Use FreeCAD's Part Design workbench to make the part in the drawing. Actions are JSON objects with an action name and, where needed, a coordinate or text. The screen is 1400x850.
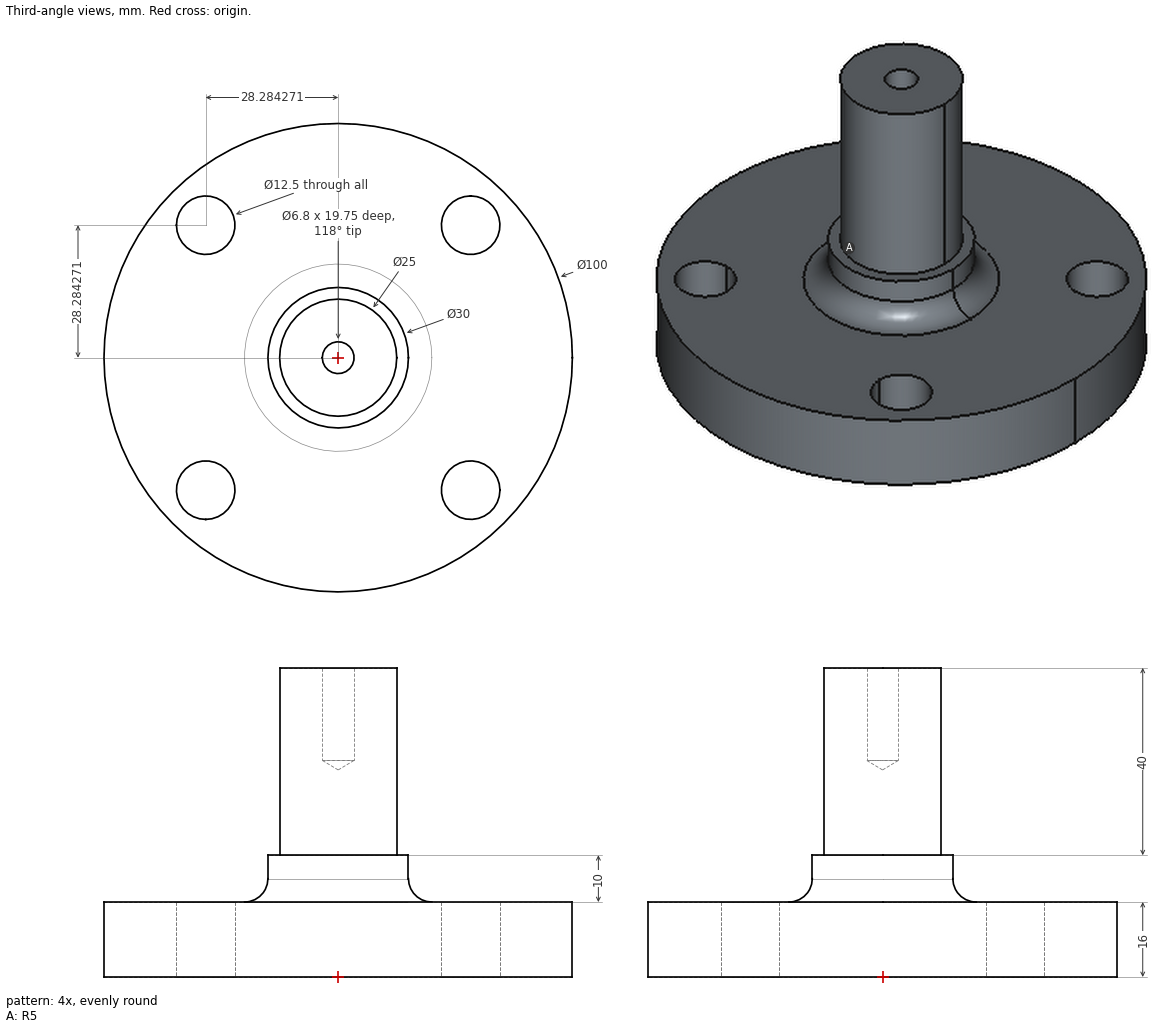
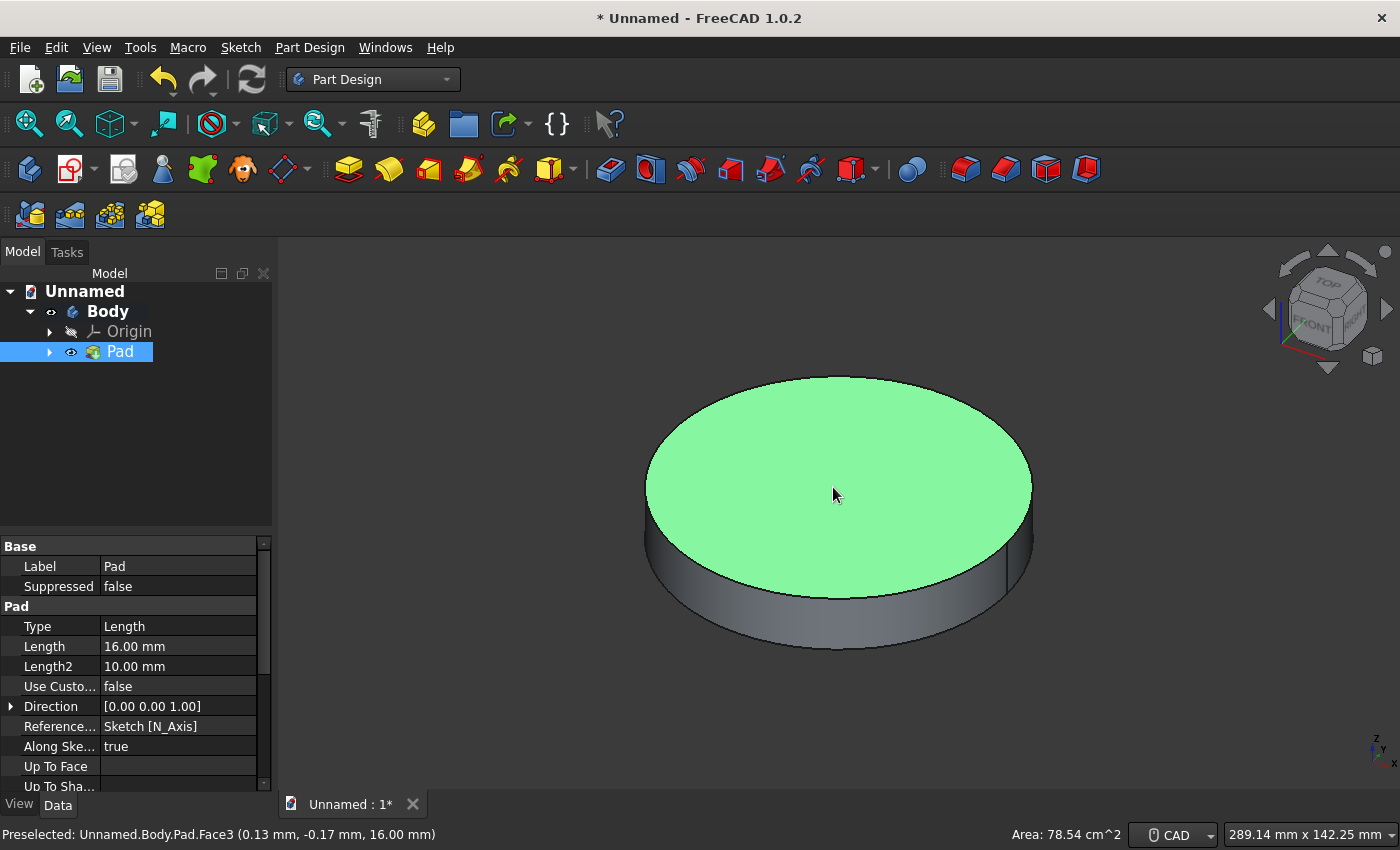
{"action": "left_click", "coordinate": [70, 170]}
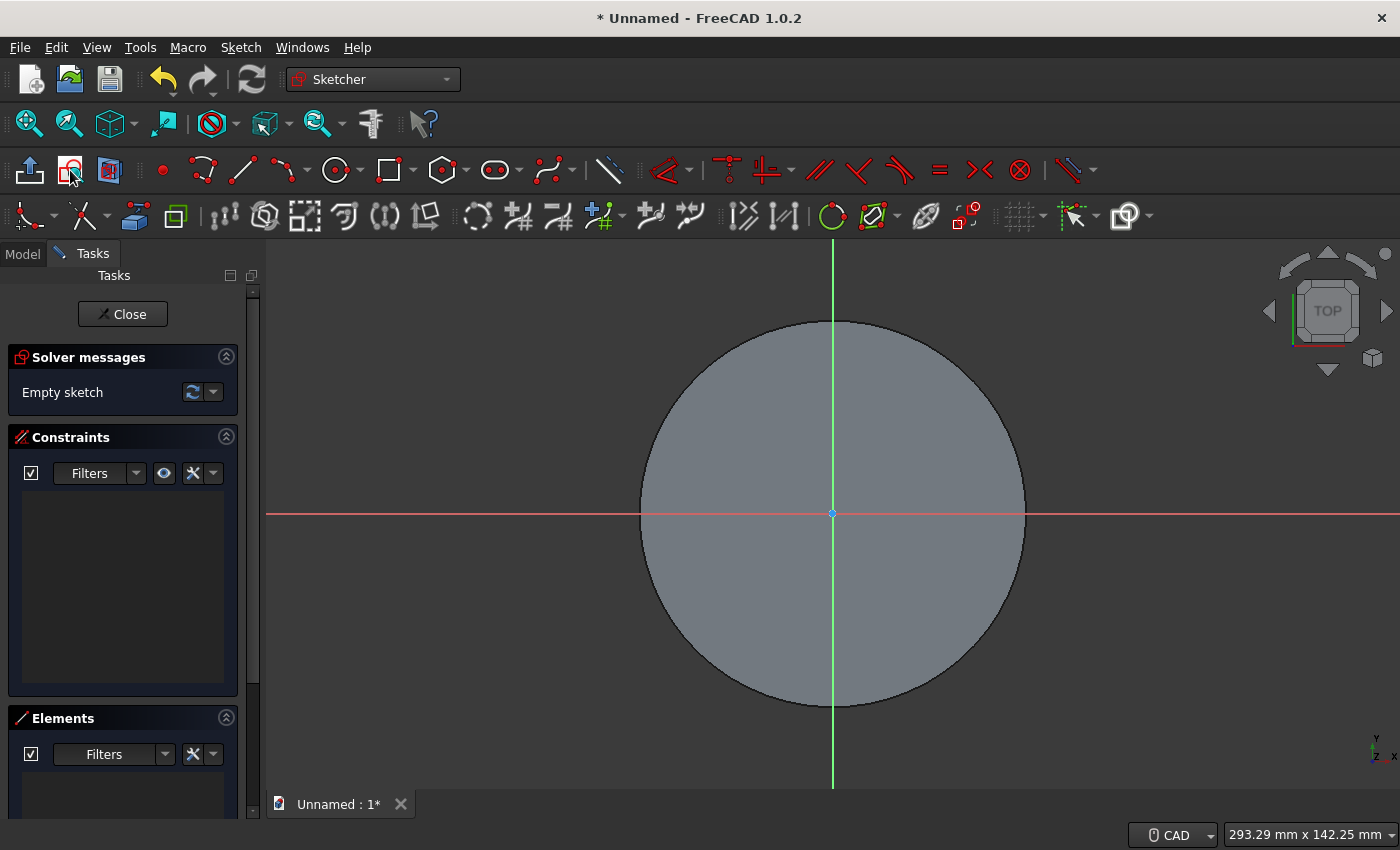
{"action": "scroll", "coordinate": [862, 514], "scroll_direction": "up", "scroll_amount": 6}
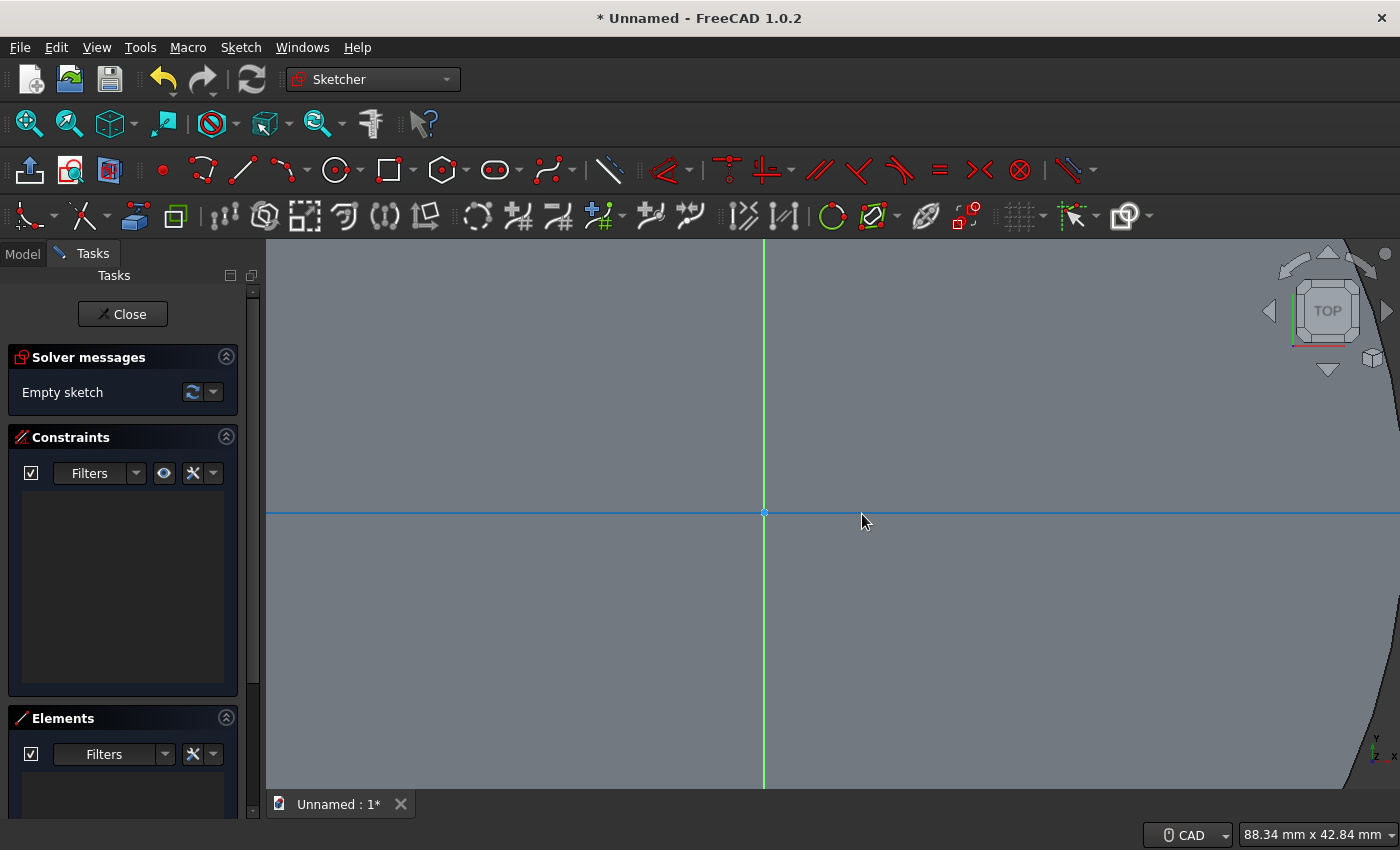
{"action": "key", "text": "g c"}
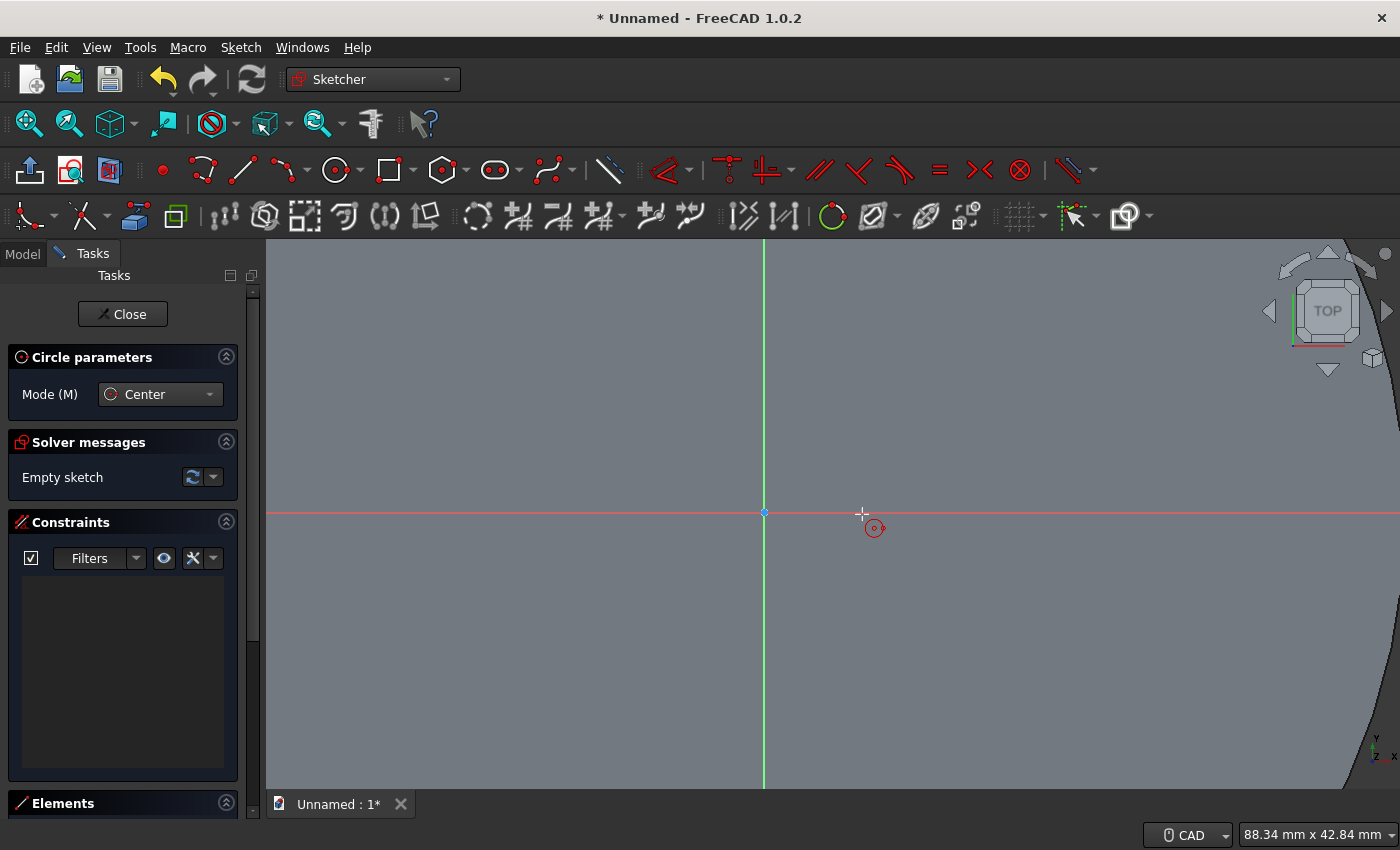
{"action": "left_click", "coordinate": [764, 513]}
{"action": "left_click", "coordinate": [900, 377]}
{"action": "key", "text": "Escape"}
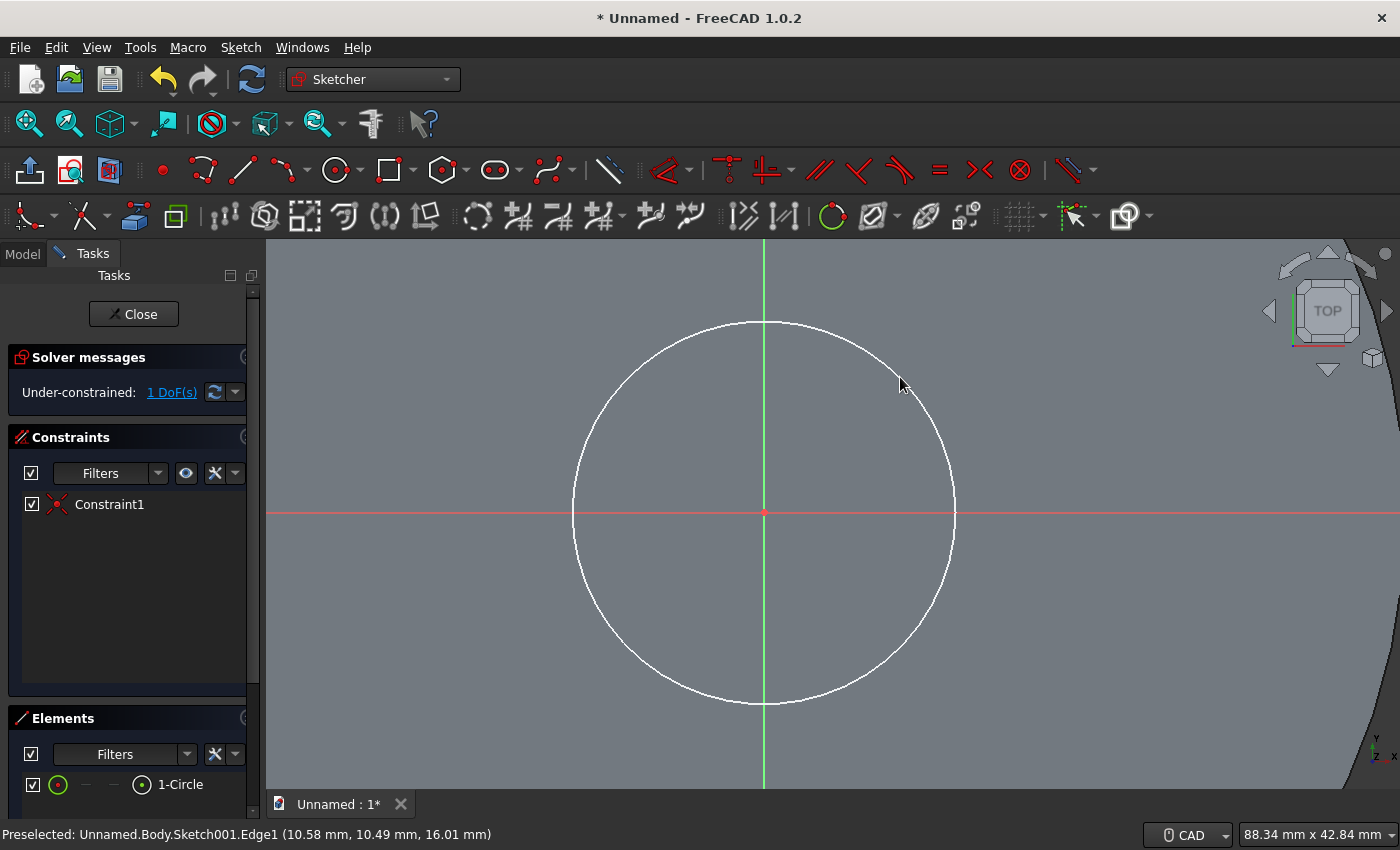
{"action": "left_click", "coordinate": [664, 170]}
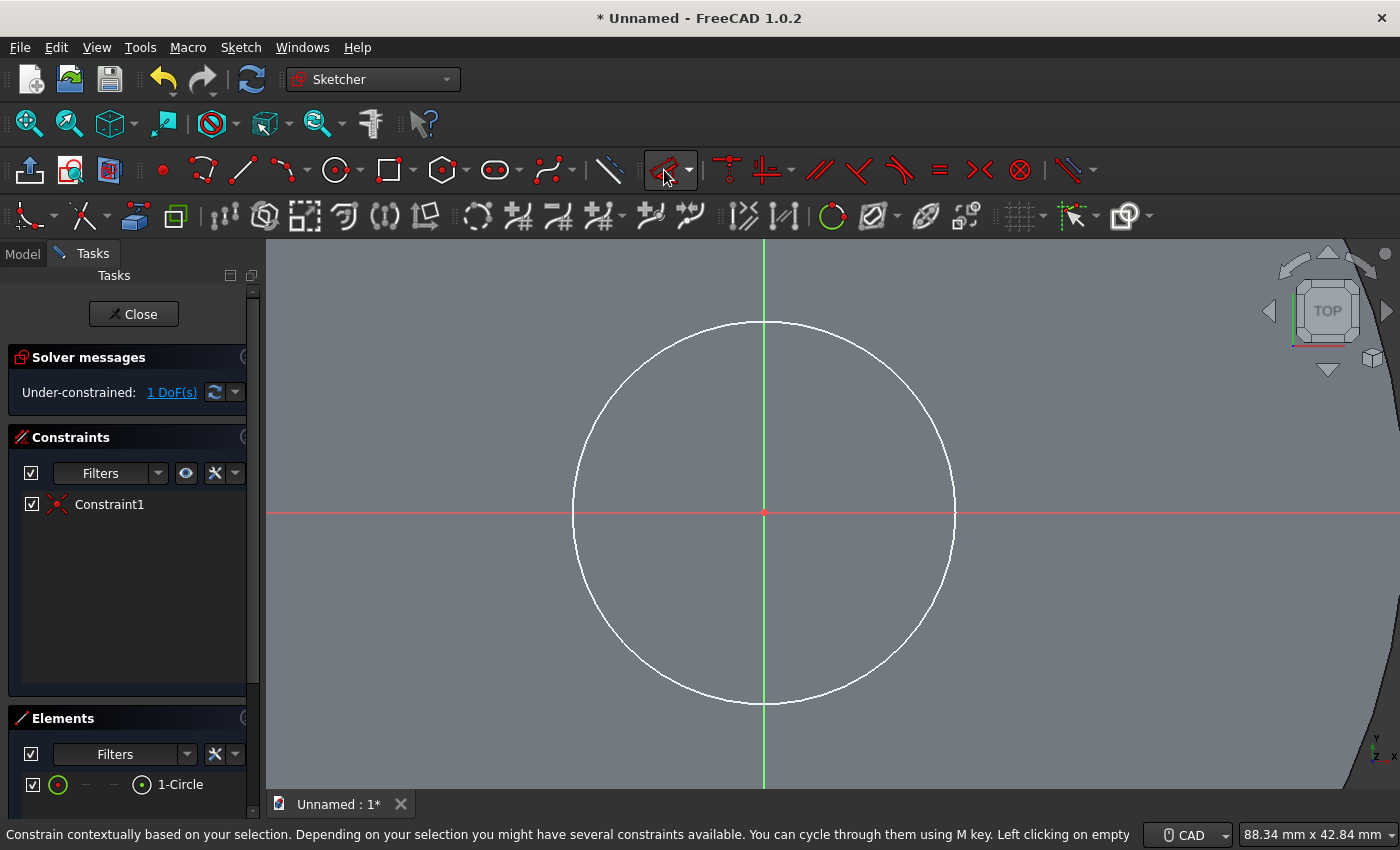
{"action": "left_click", "coordinate": [899, 377]}
{"action": "left_click", "coordinate": [922, 354]}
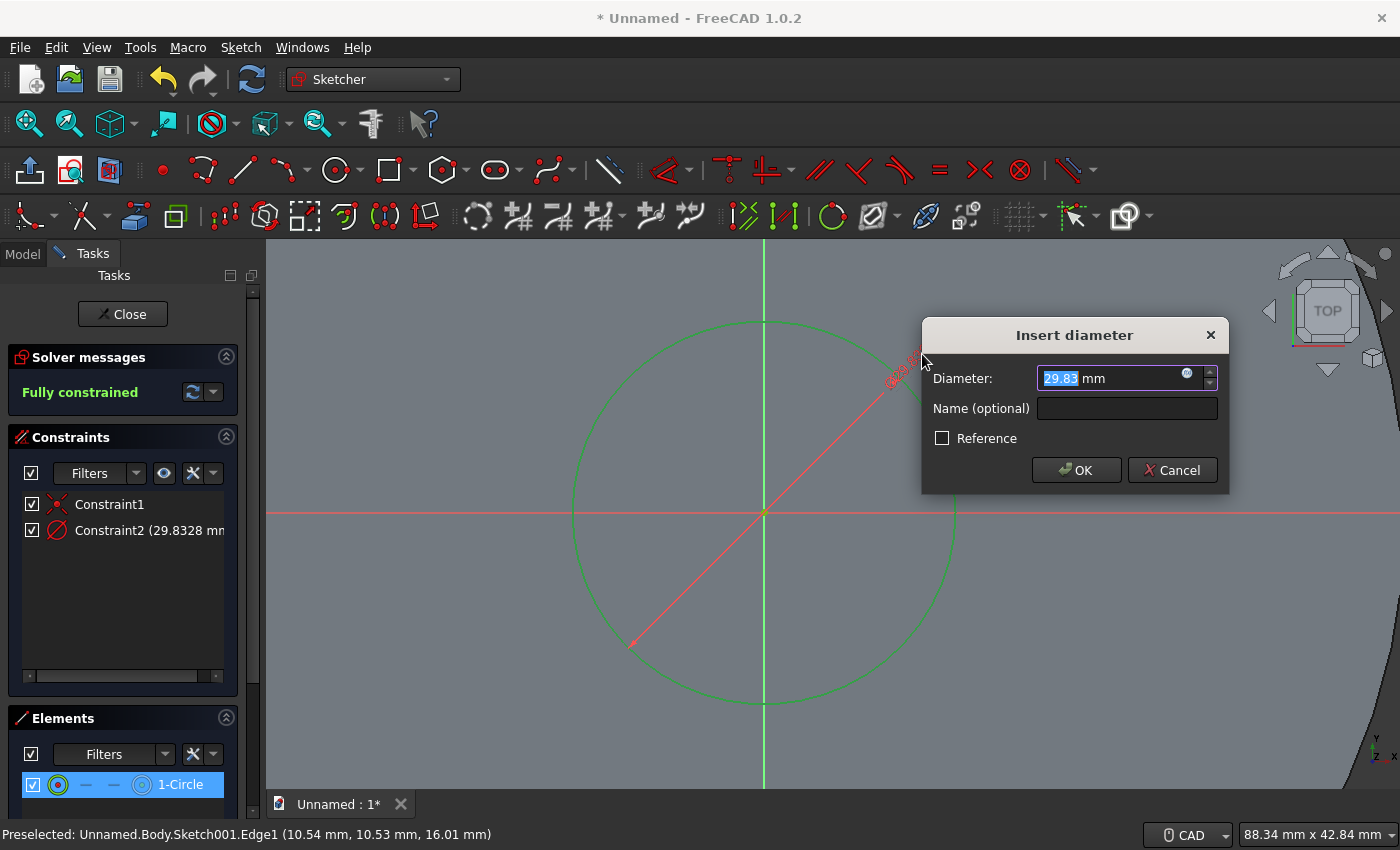
{"action": "type", "text": "30"}
{"action": "key", "text": "Return"}
{"action": "key", "text": "Escape"}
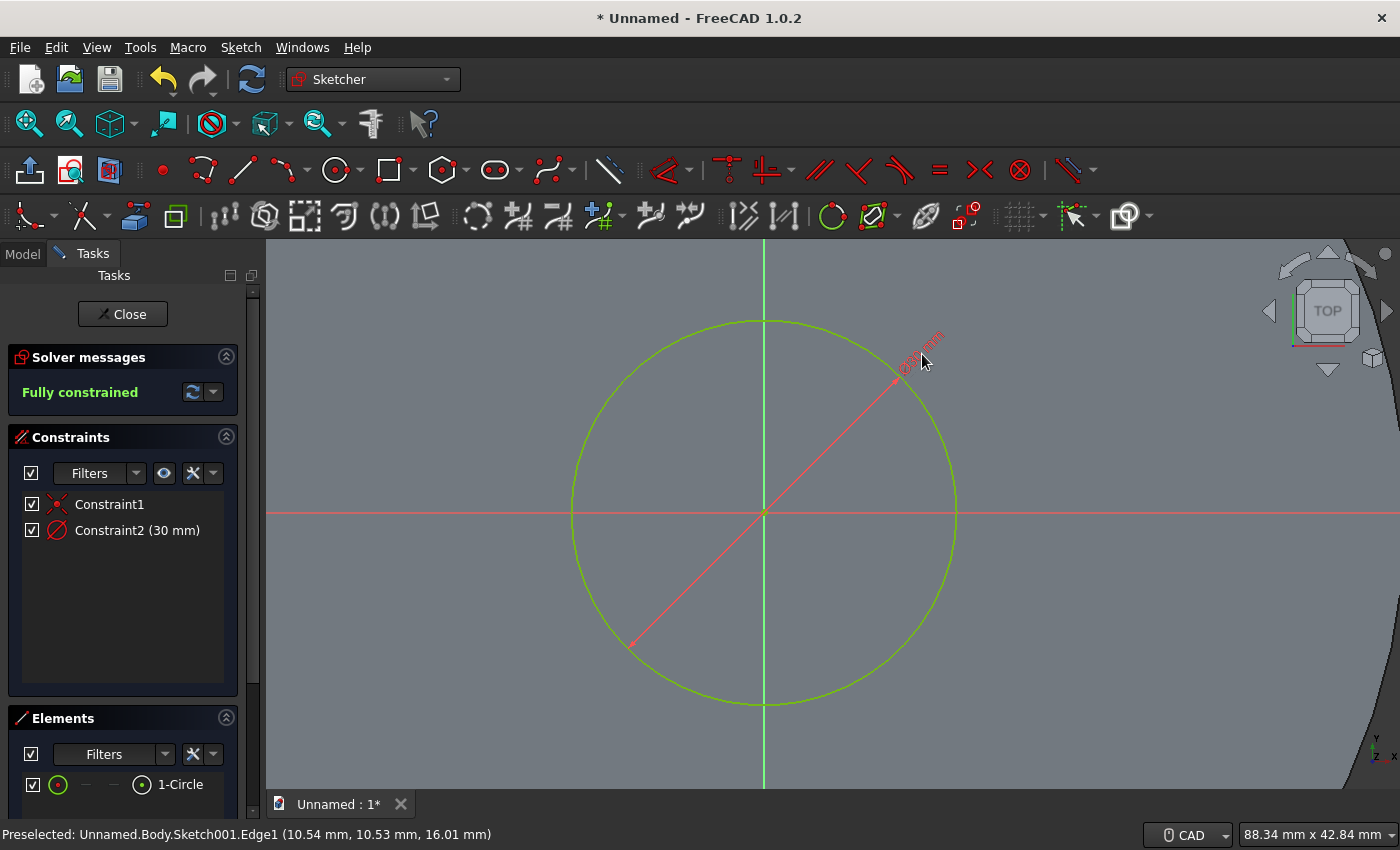
{"action": "left_click", "coordinate": [123, 314]}